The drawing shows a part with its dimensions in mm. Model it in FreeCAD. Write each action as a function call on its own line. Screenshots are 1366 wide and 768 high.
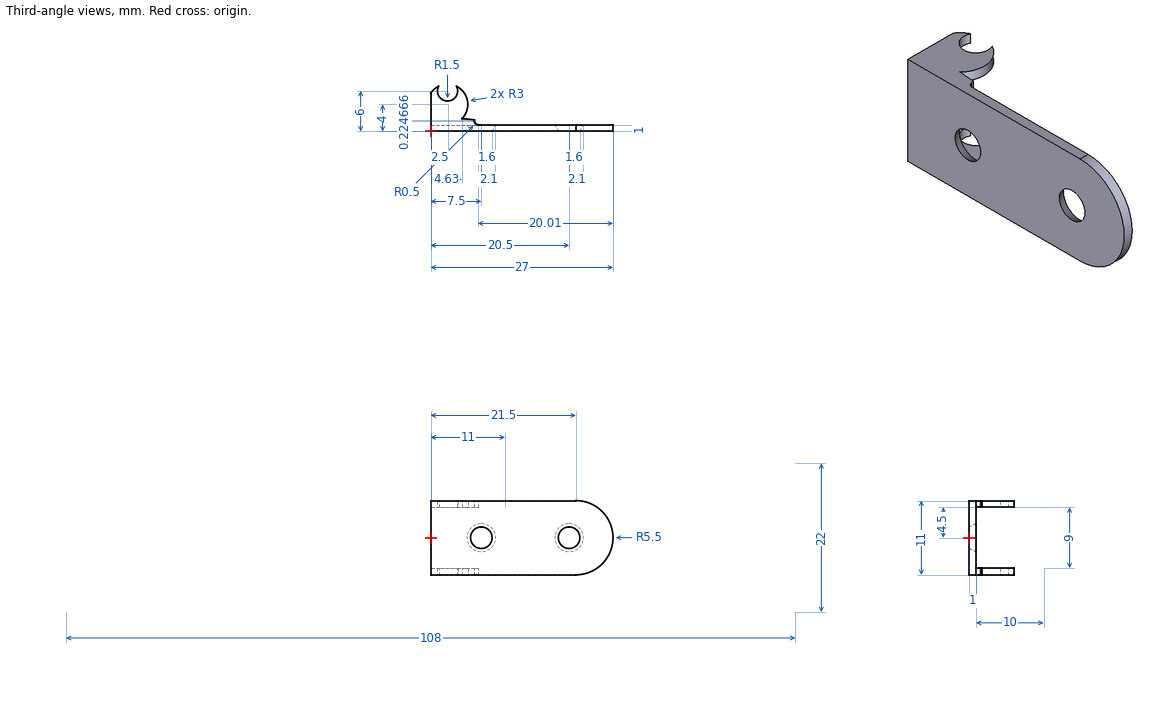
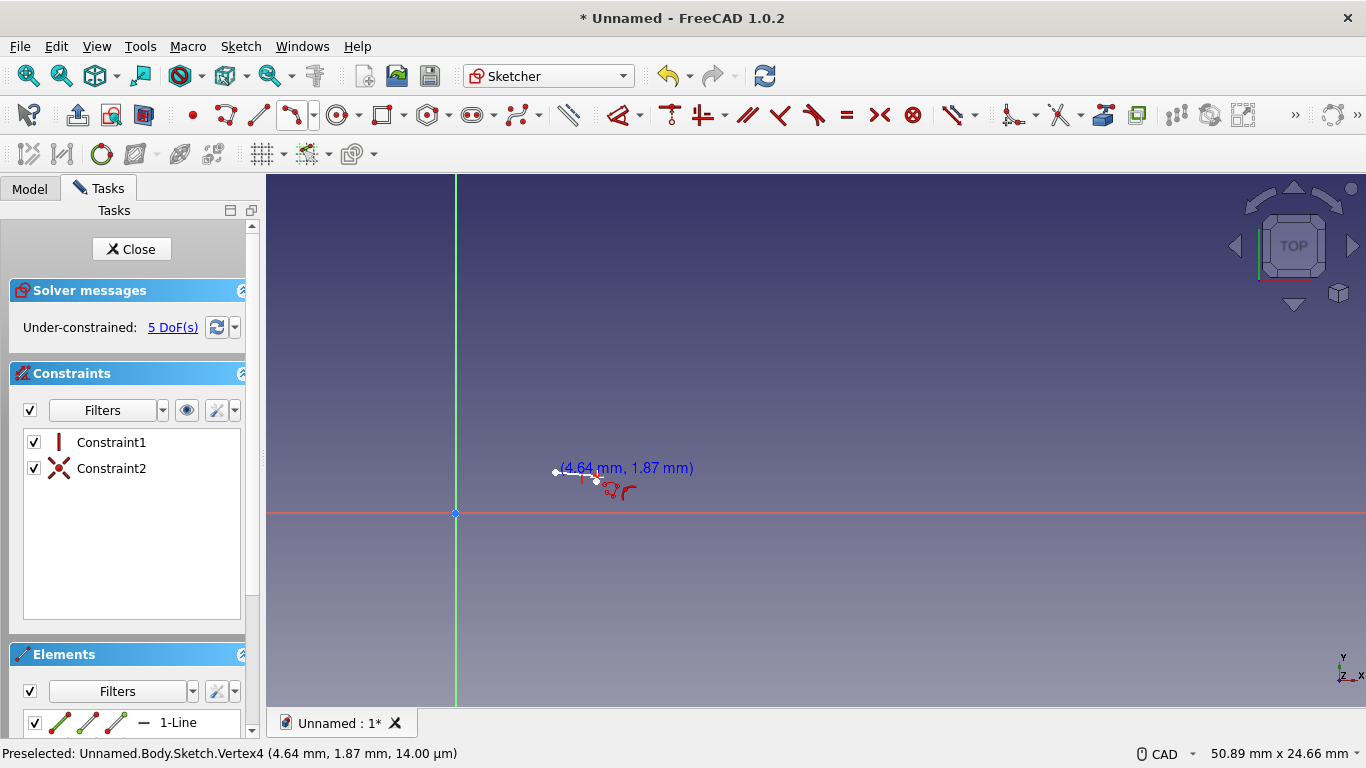
click(456, 391)
click(456, 513)
click(1039, 504)
click(1039, 491)
click(607, 491)
right_click(607, 491)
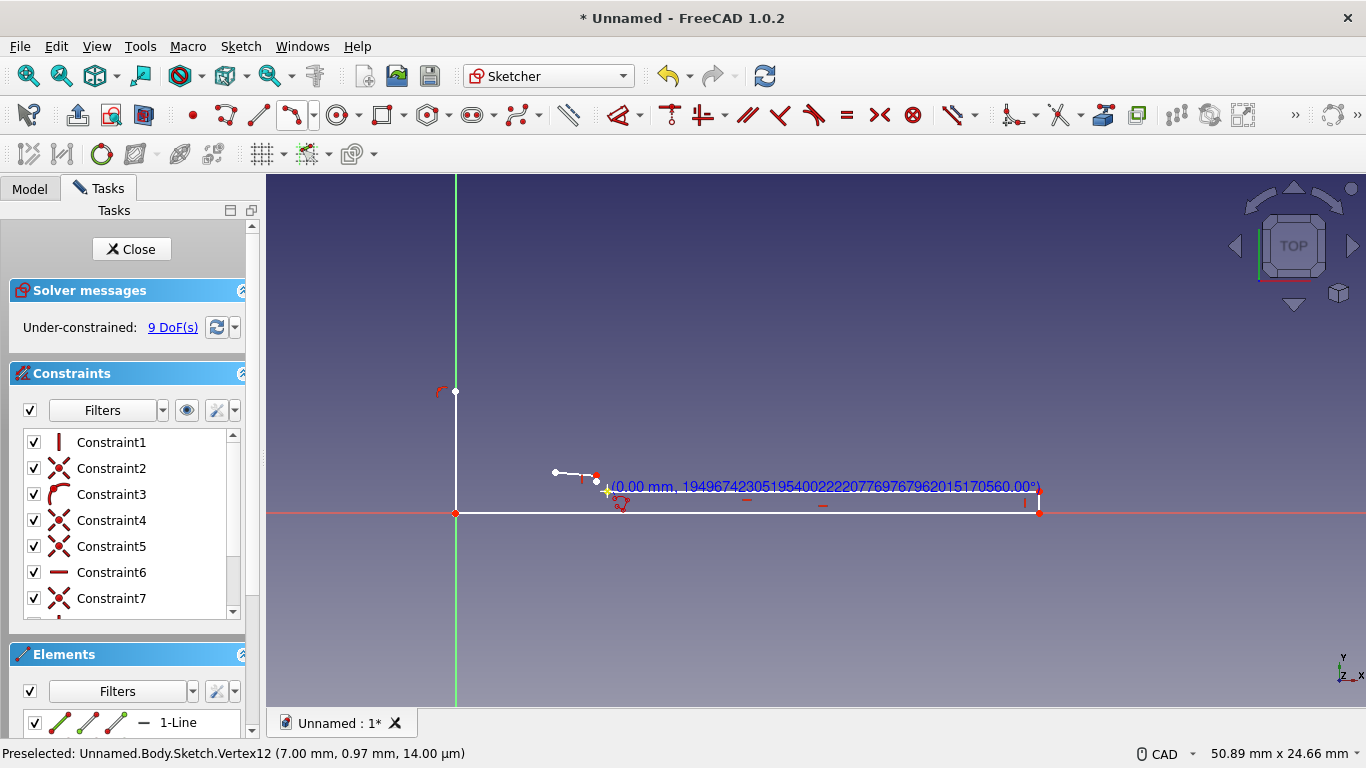
key(g)
key(3)
key(a)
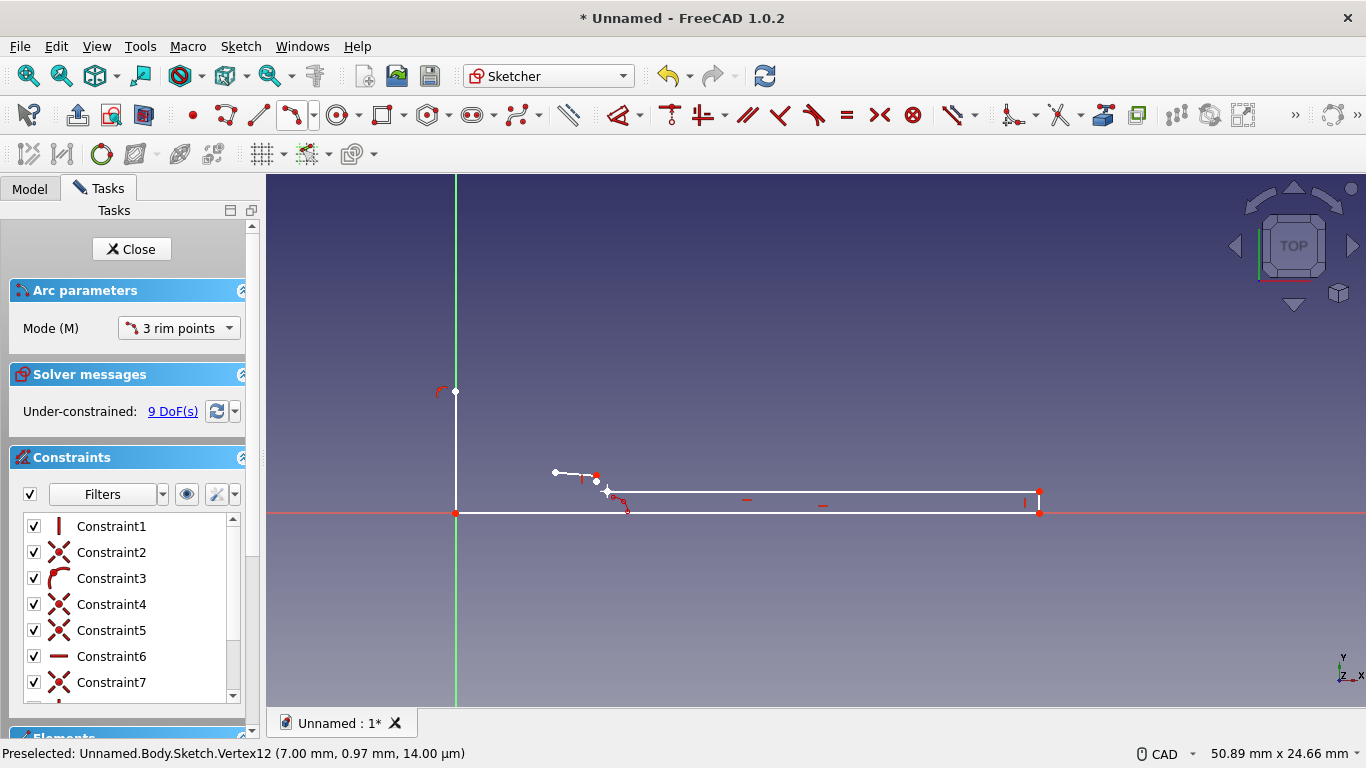
click(556, 473)
click(539, 368)
click(574, 416)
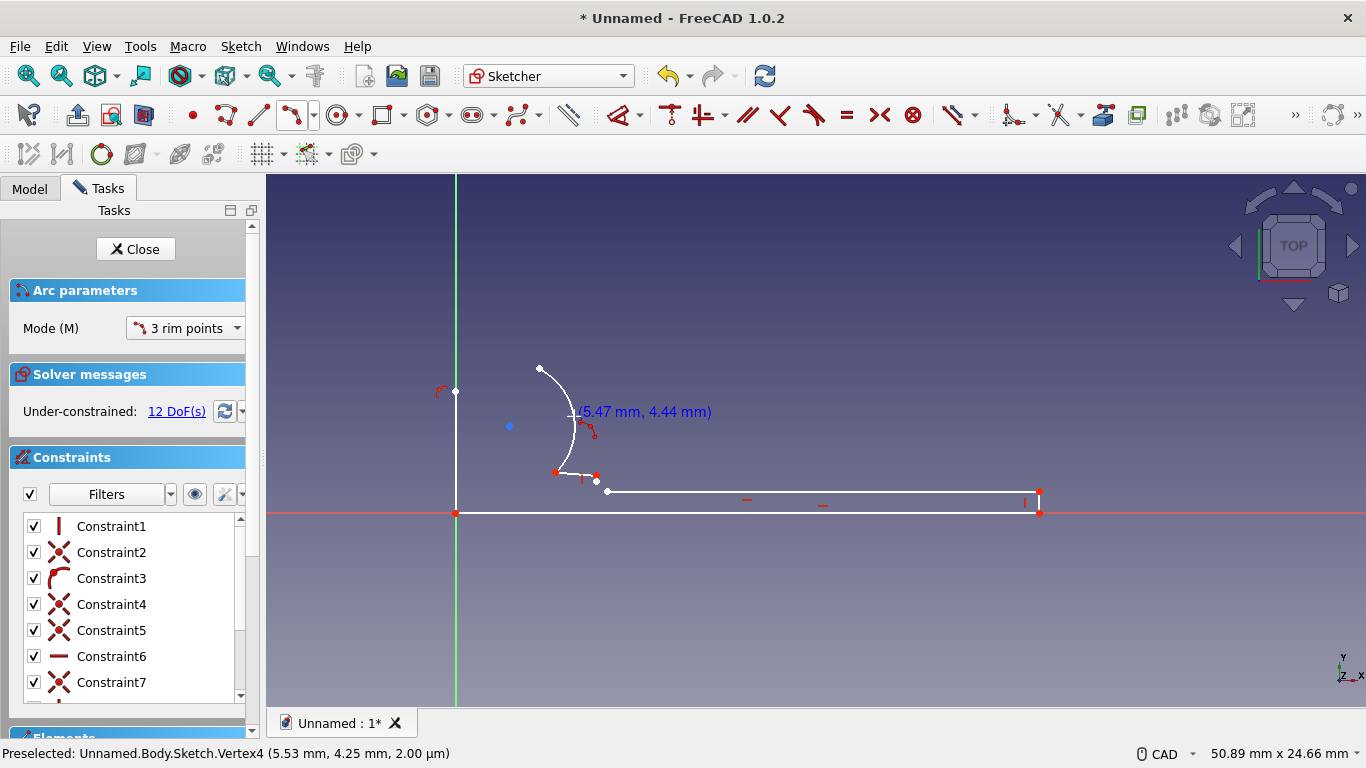
click(539, 369)
click(481, 368)
click(497, 413)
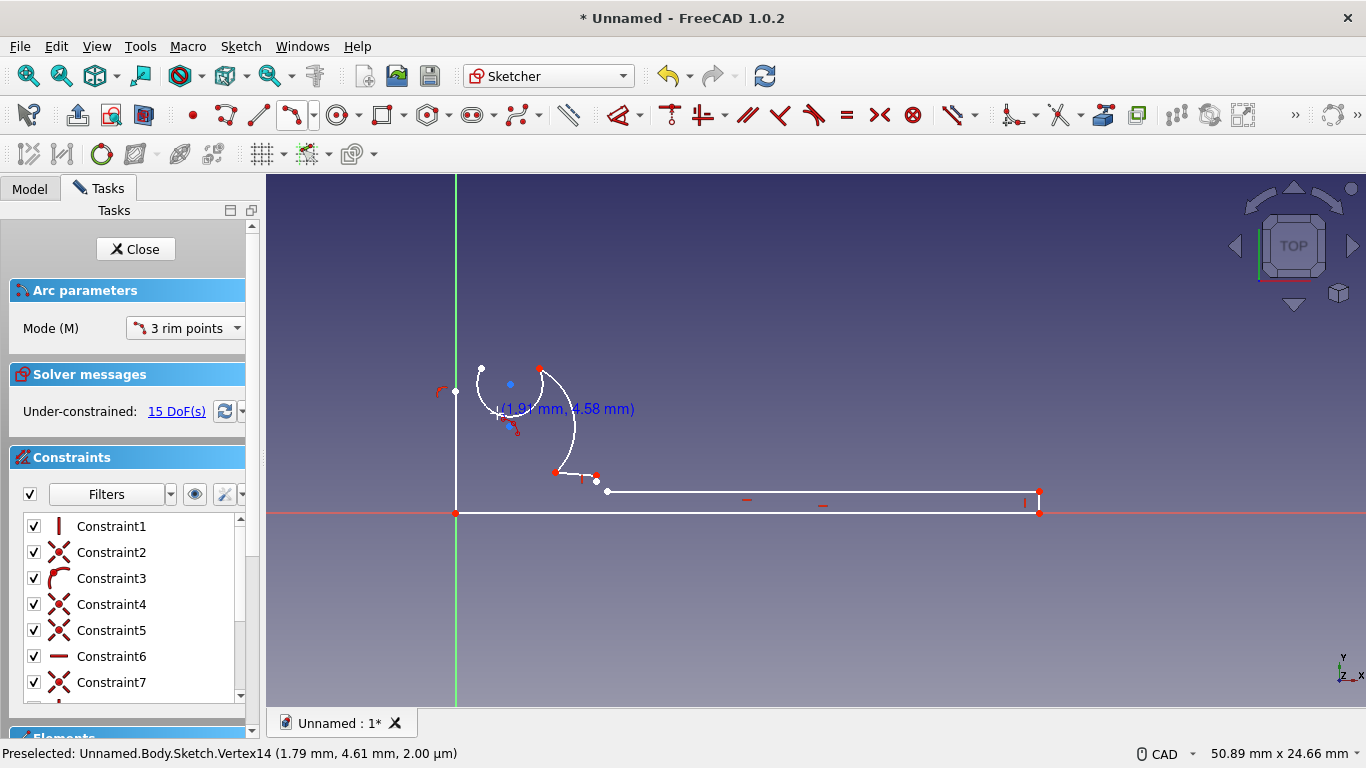
click(481, 369)
click(456, 392)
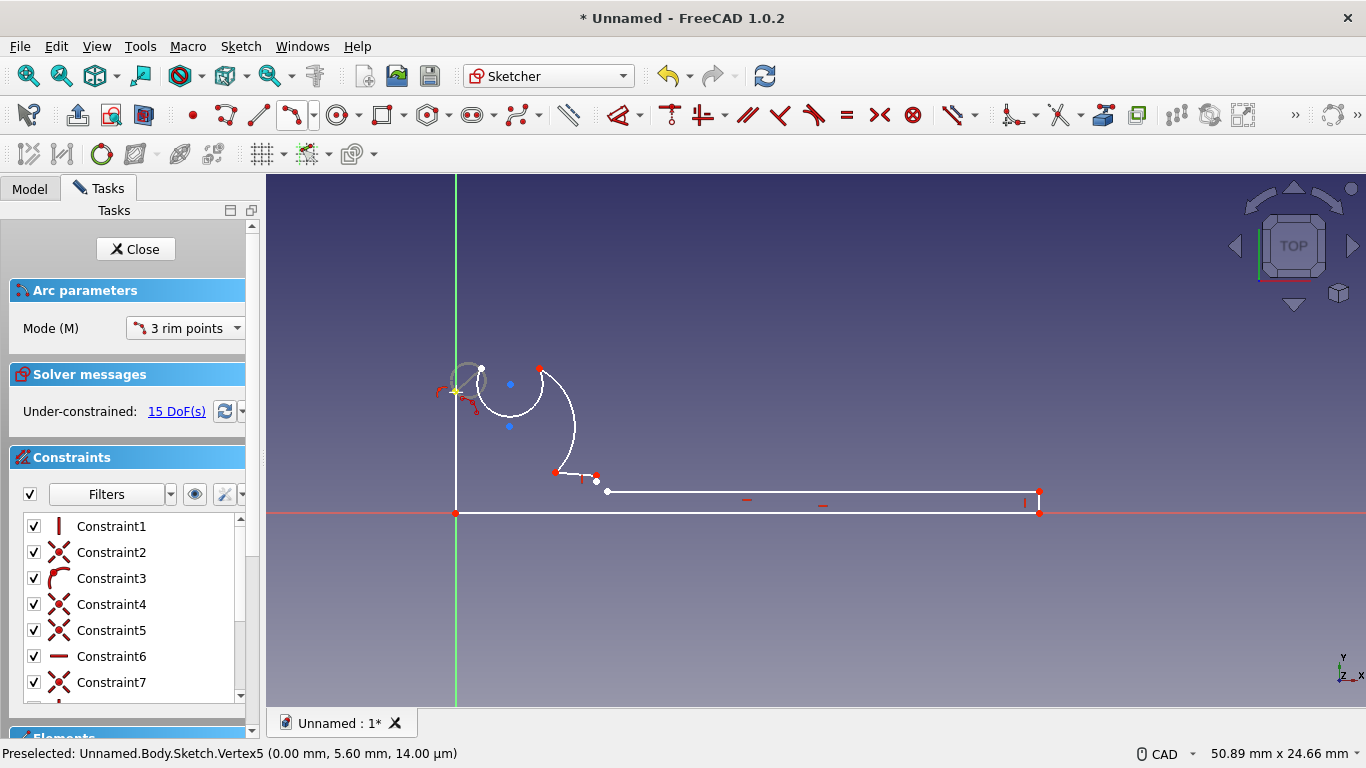
scroll(467, 378, up, 10)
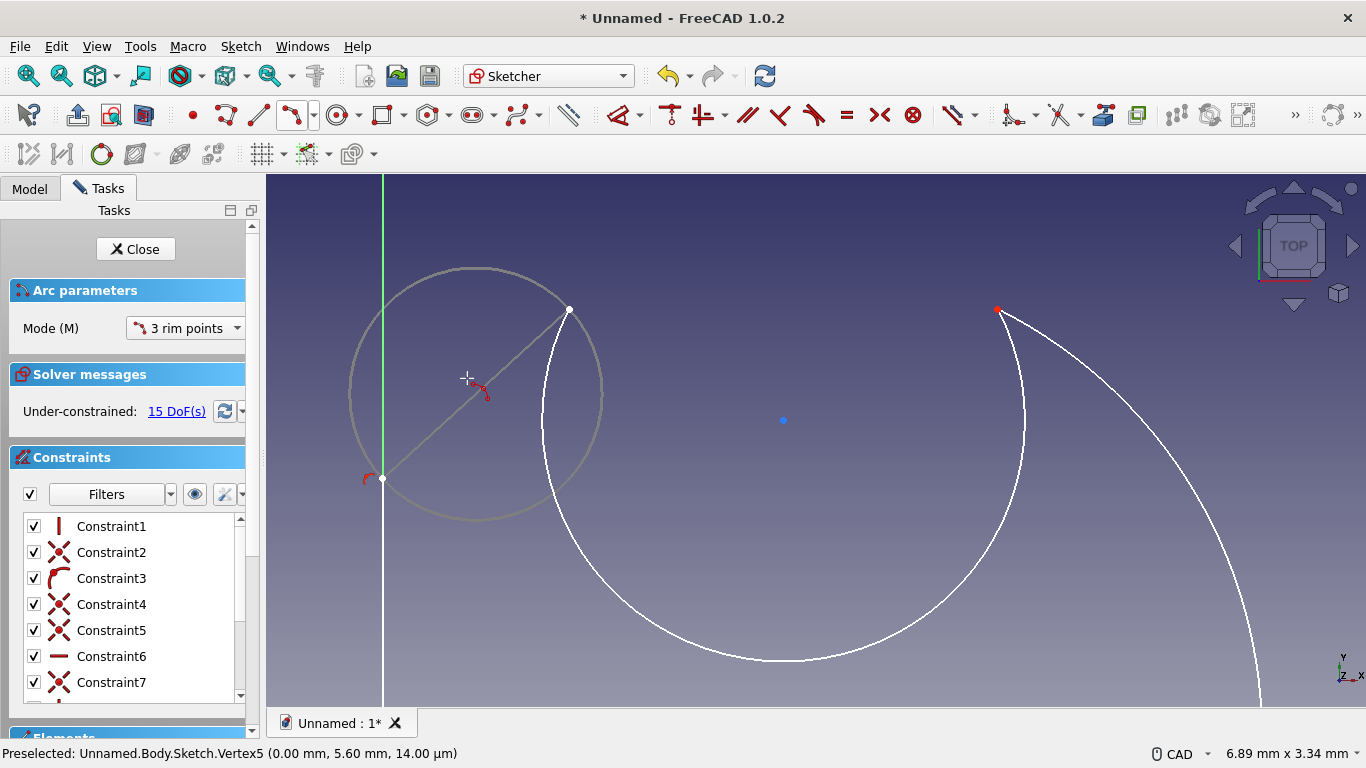
click(465, 375)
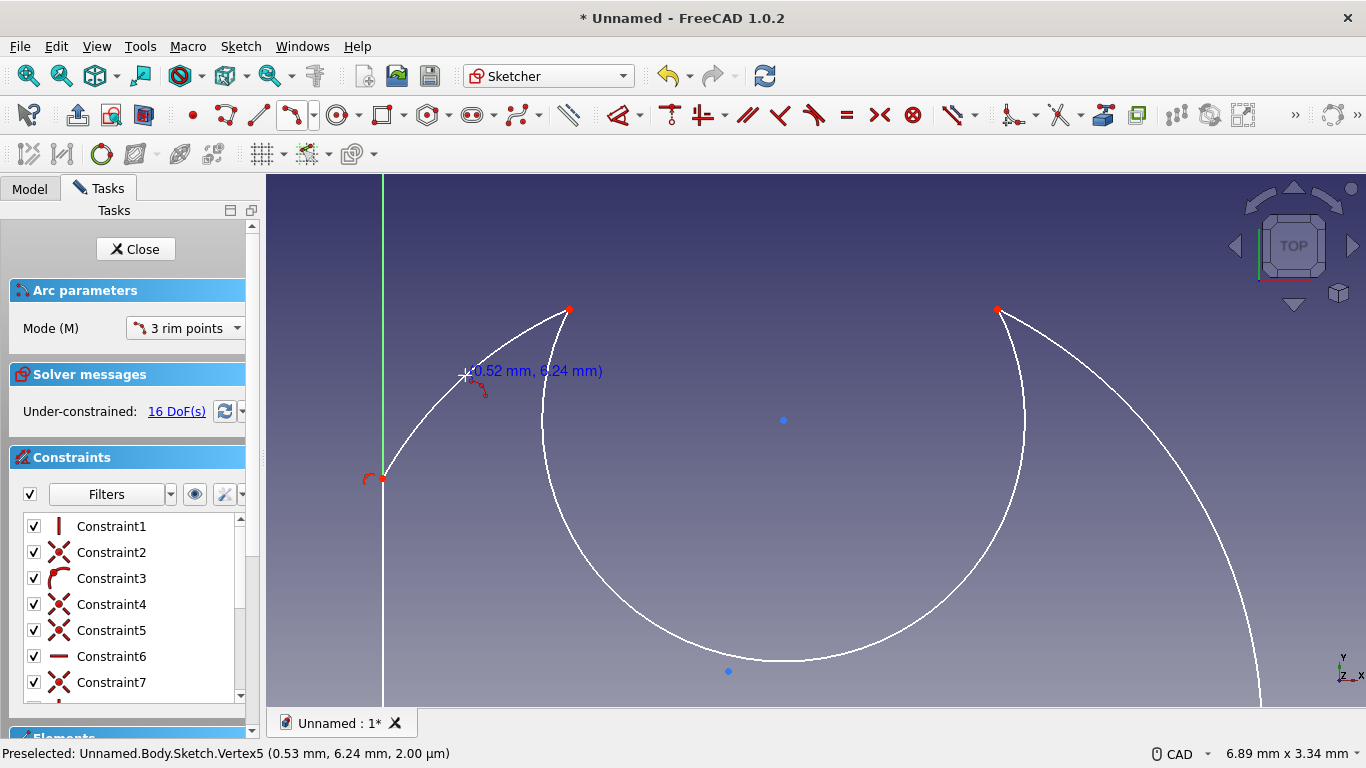
scroll(467, 378, down, 10)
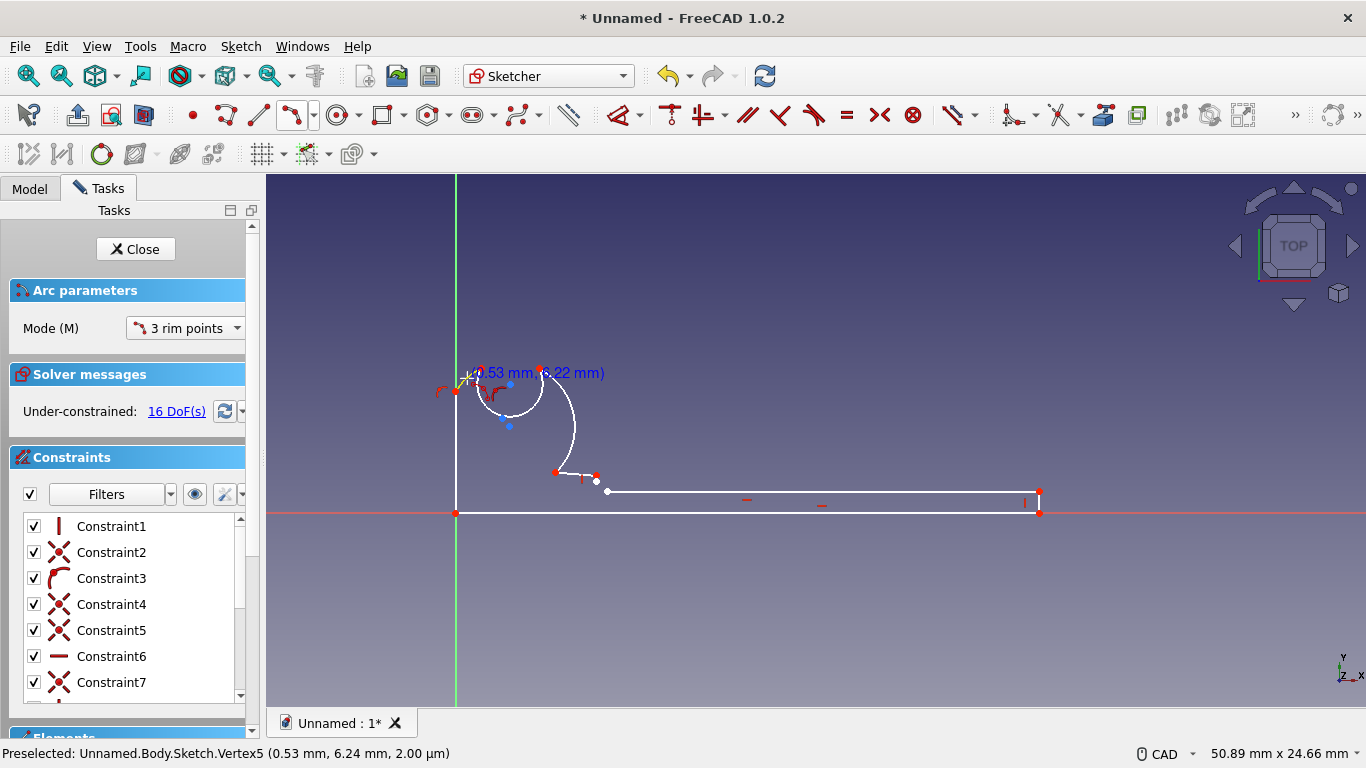
click(607, 492)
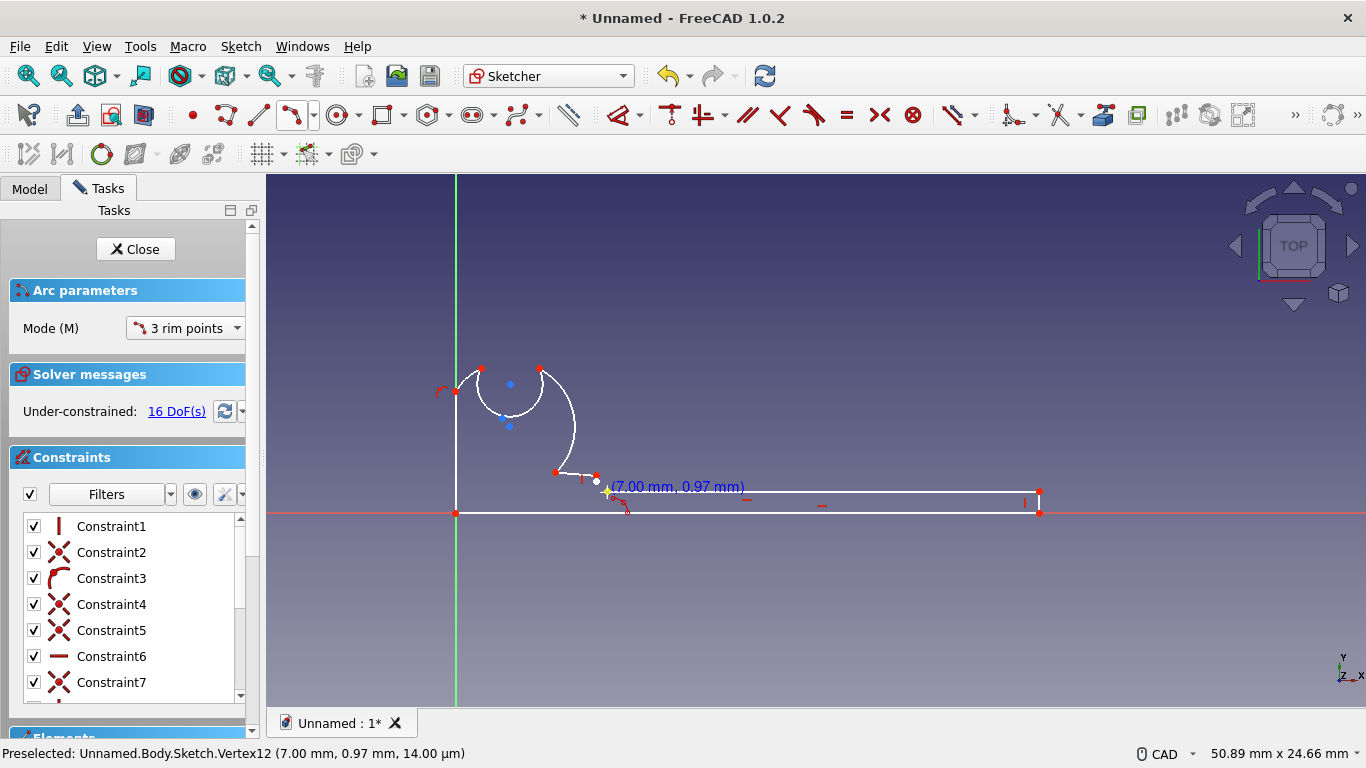
scroll(596, 481, up, 10)